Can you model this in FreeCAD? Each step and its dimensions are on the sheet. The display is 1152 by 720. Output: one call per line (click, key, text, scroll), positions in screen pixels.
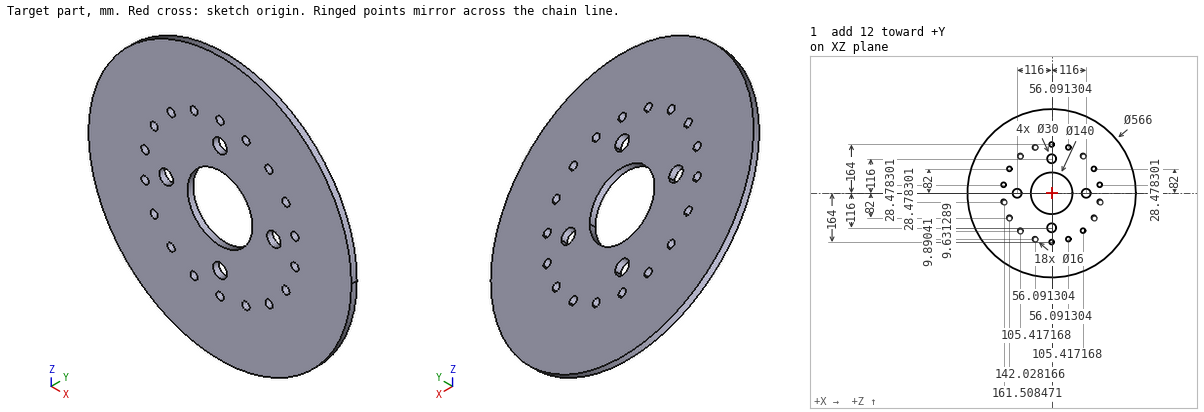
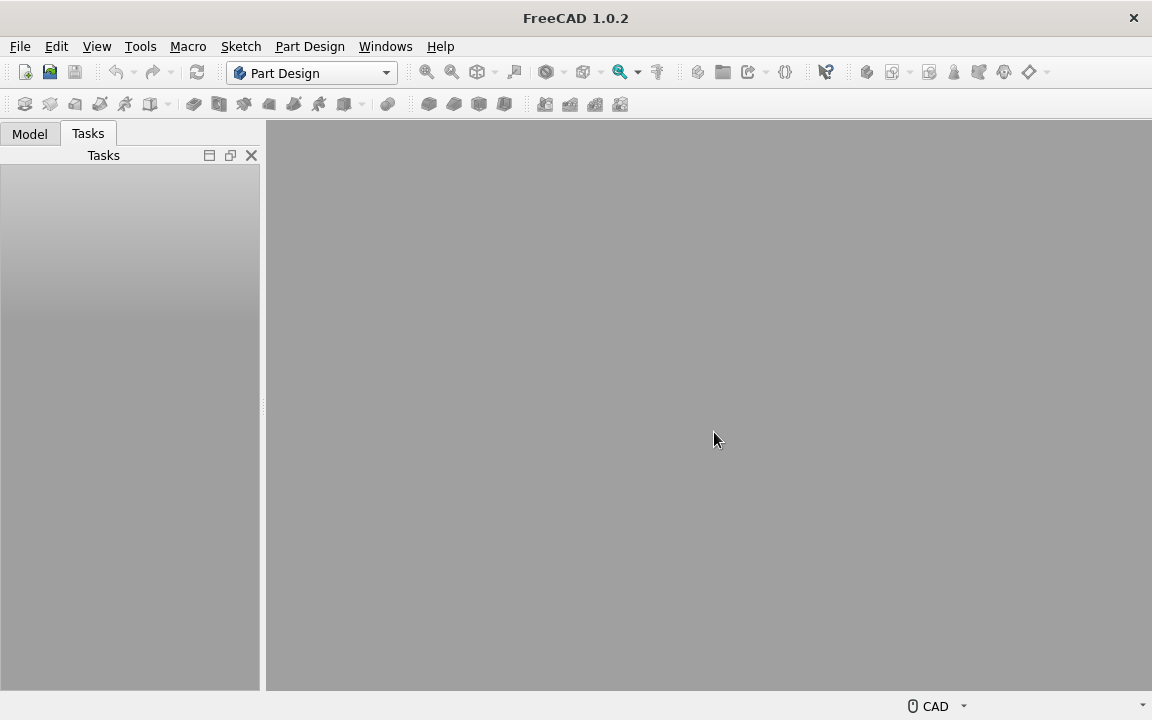
click(25, 72)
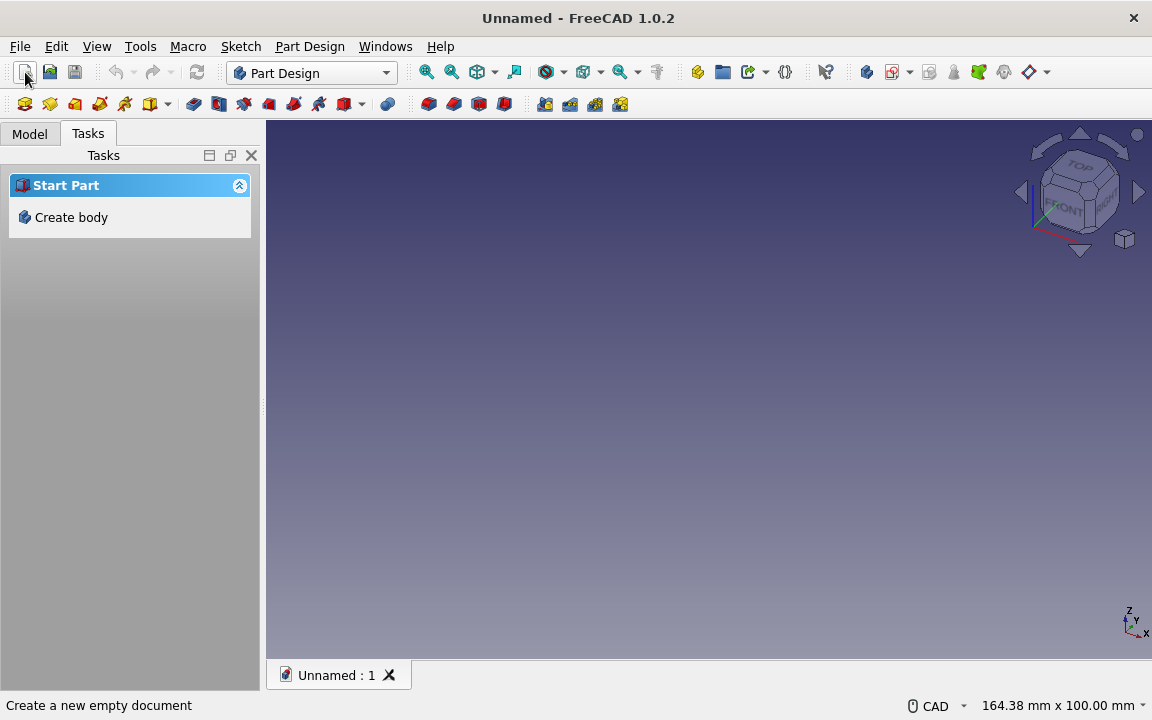
click(892, 72)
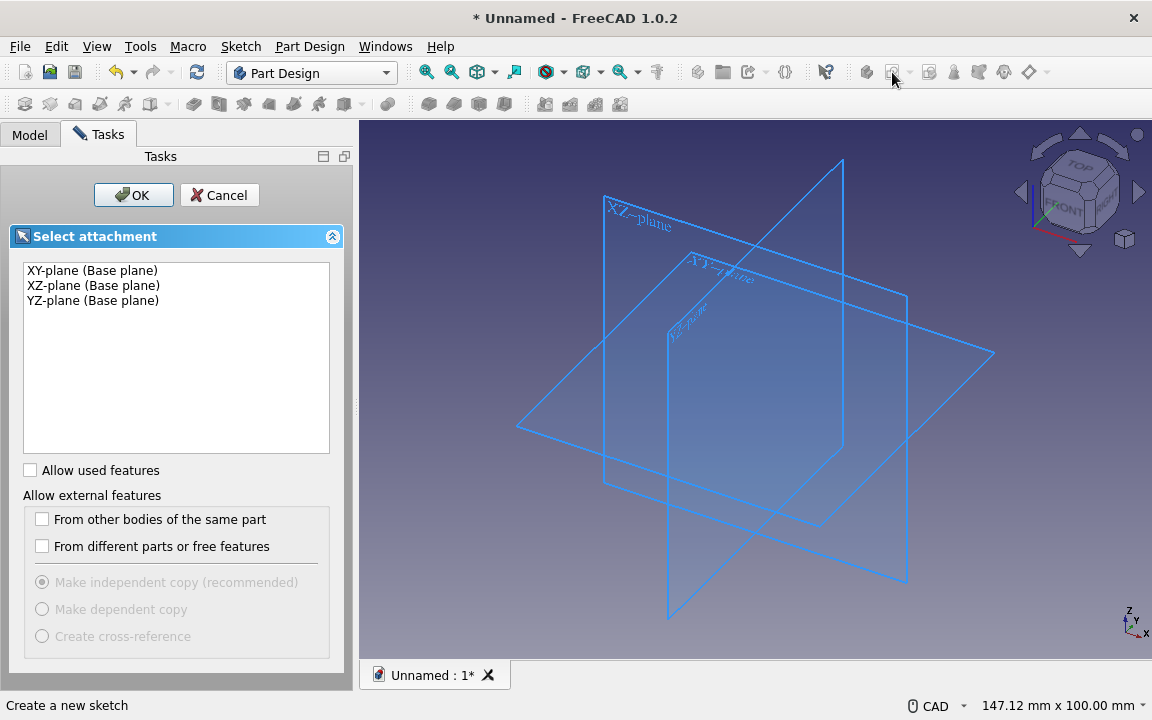
click(84, 286)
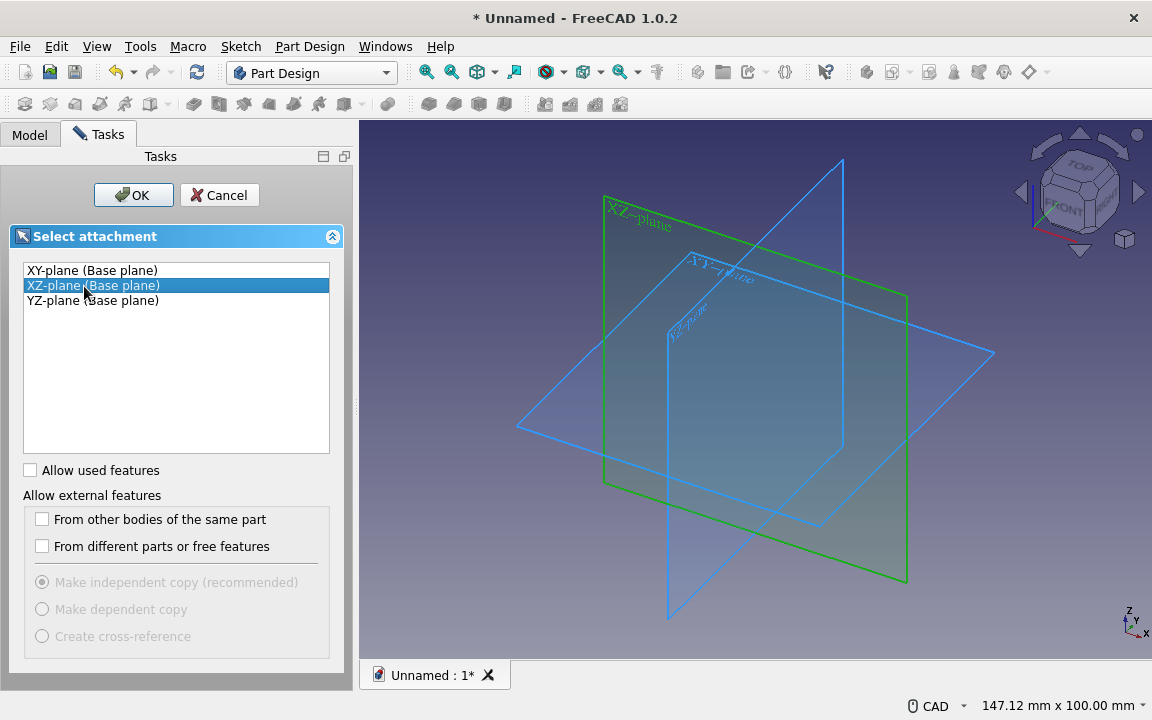
click(134, 195)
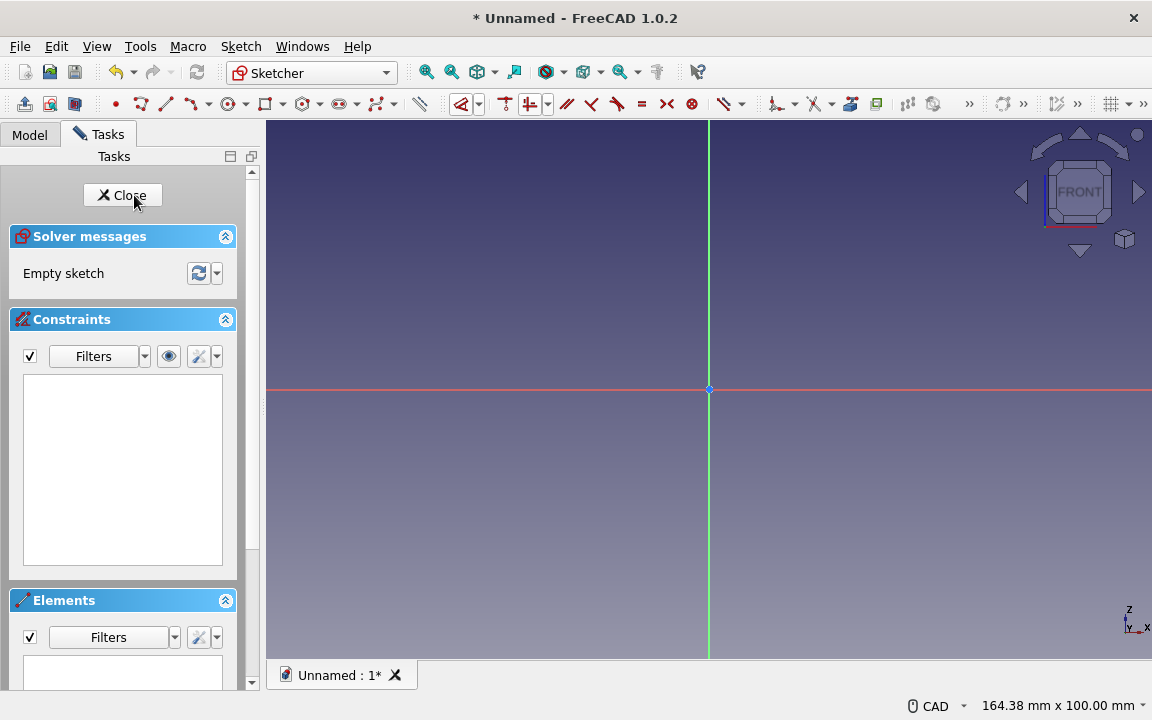
scroll(632, 390, down, 11)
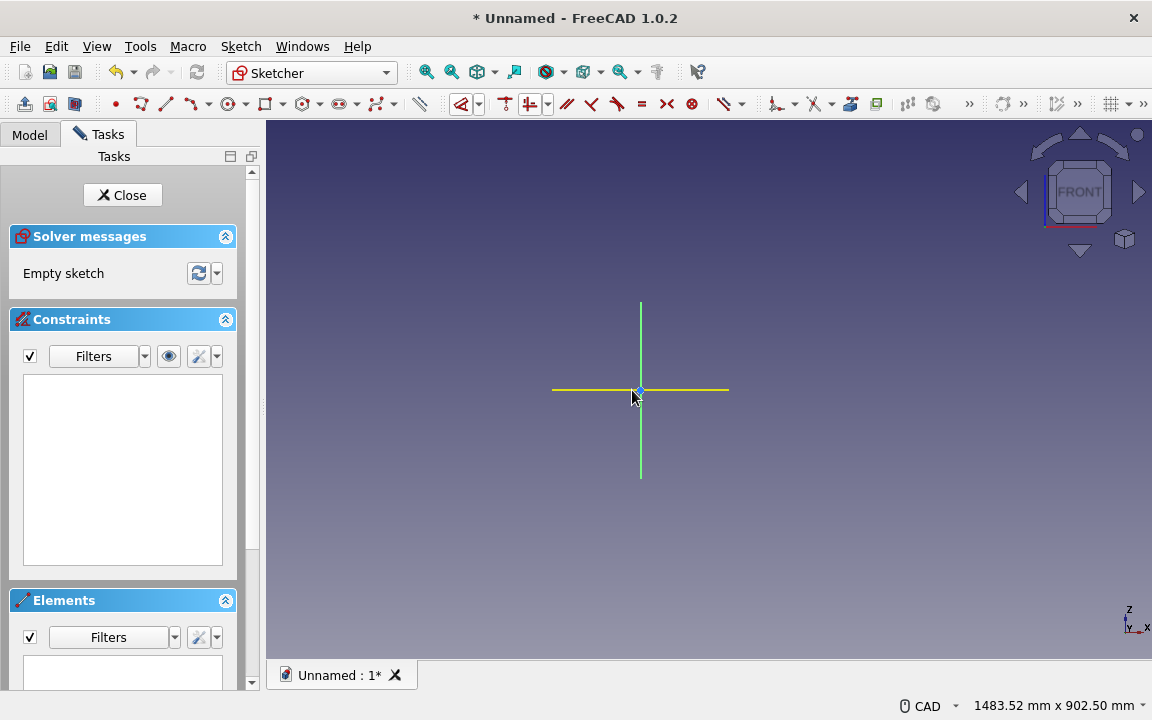
key(g)
key(c)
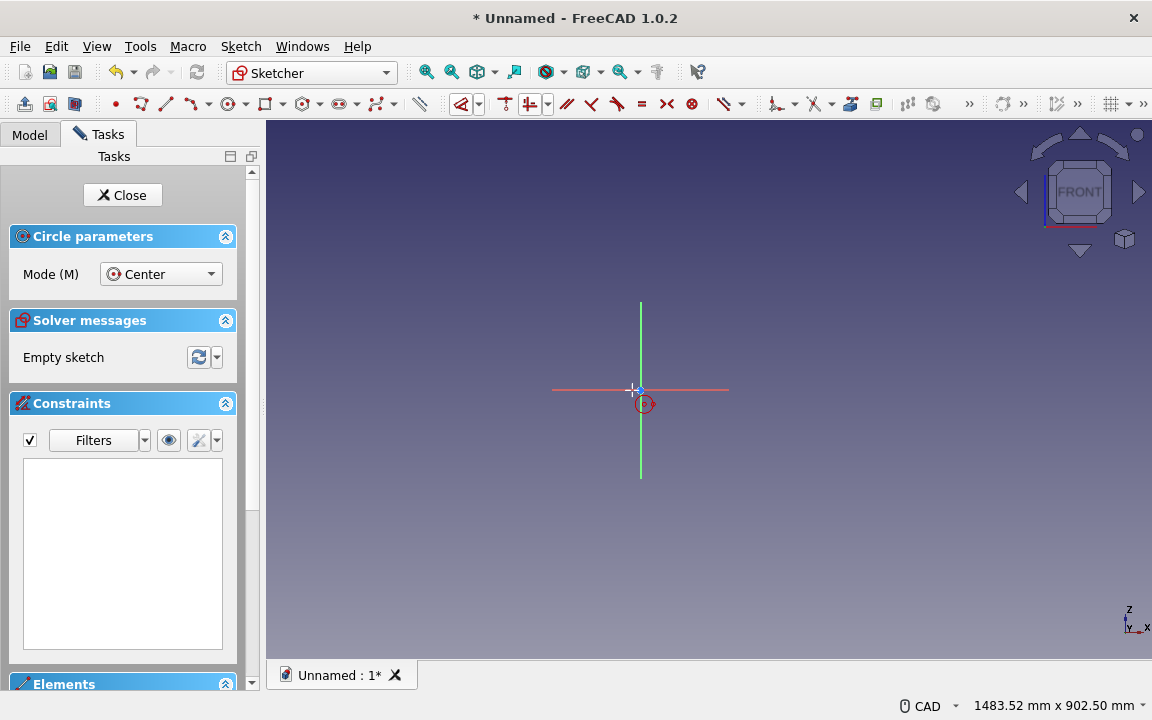
click(641, 390)
move(760, 271)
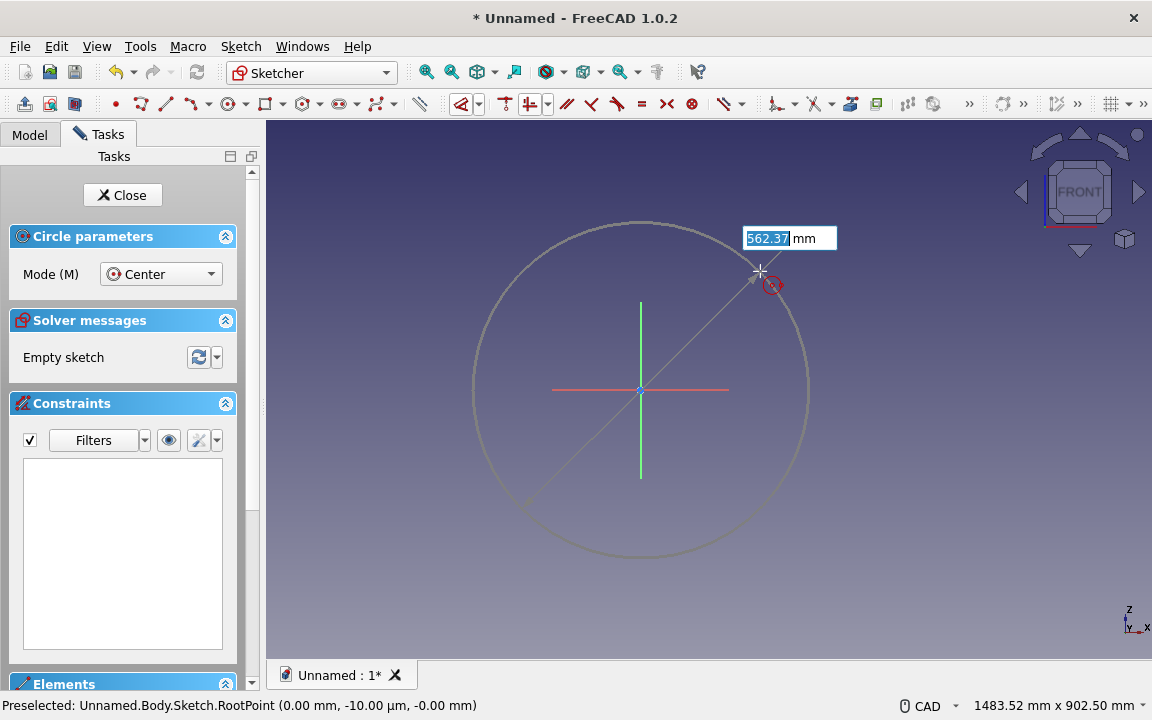
text(566)
key(Return)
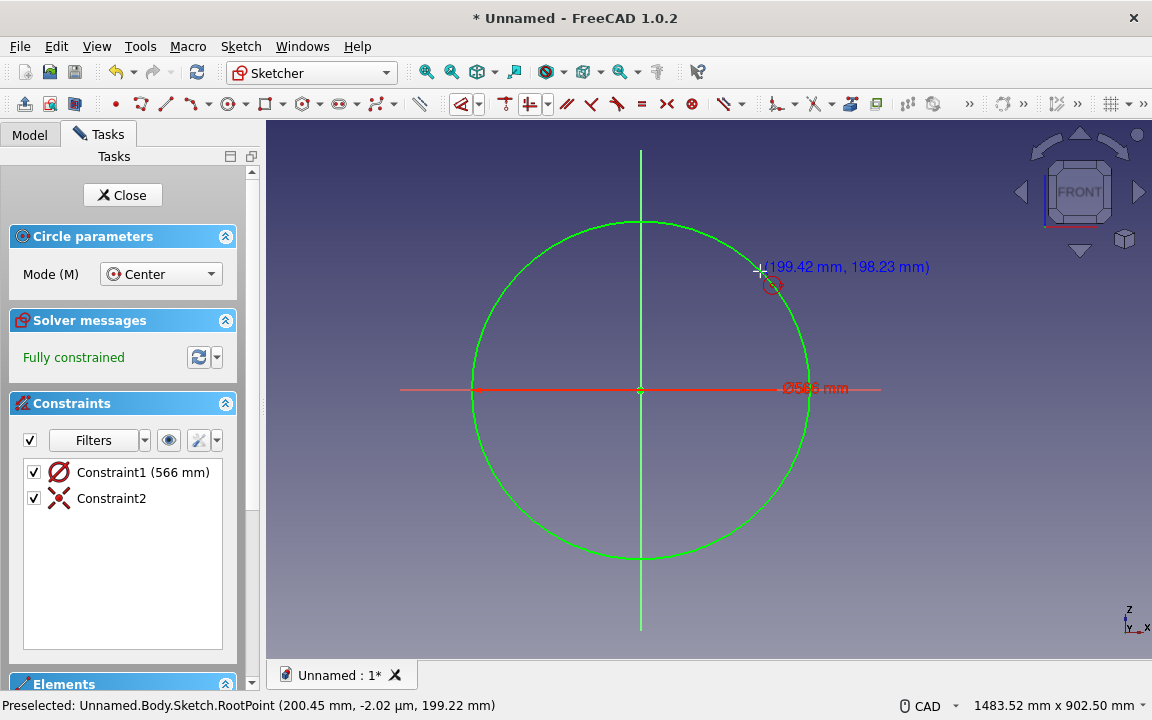
scroll(578, 465, up, 8)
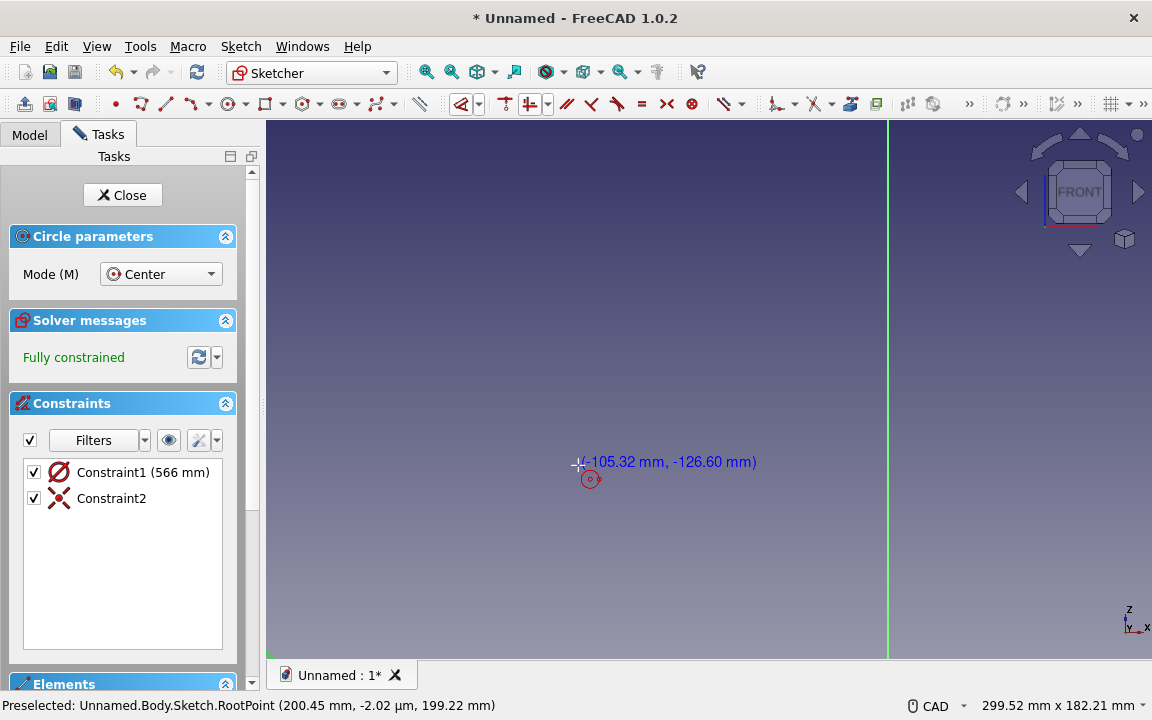
scroll(578, 465, down, 8)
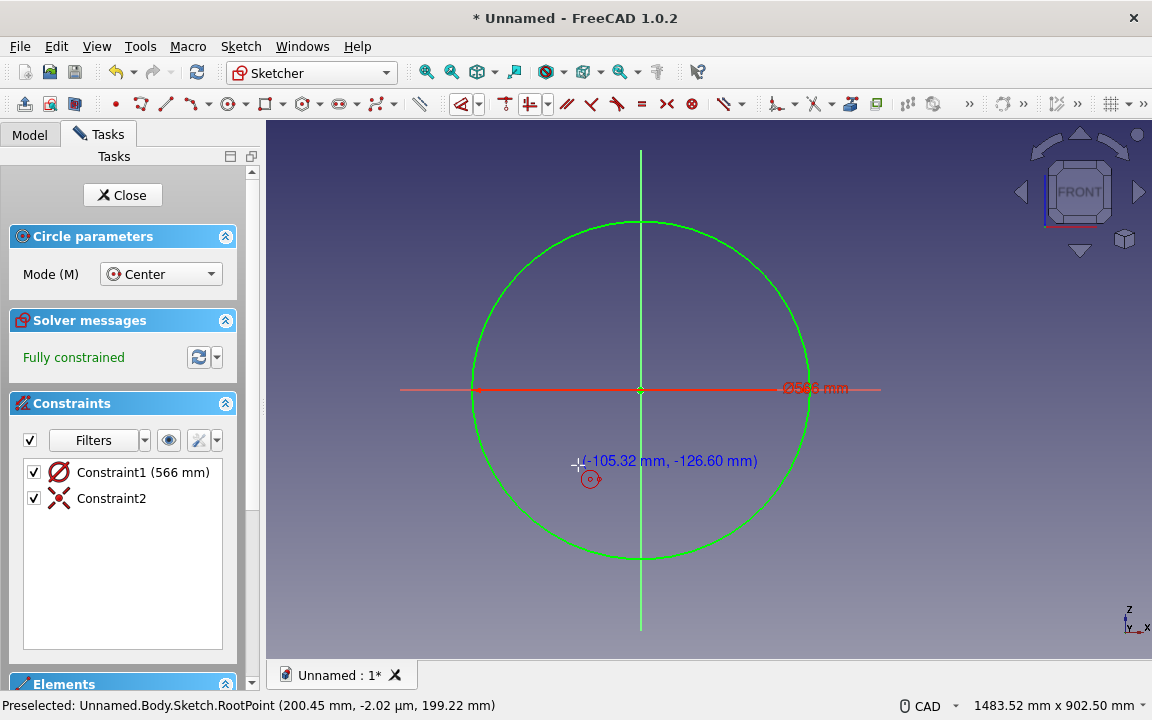
click(578, 465)
move(581, 462)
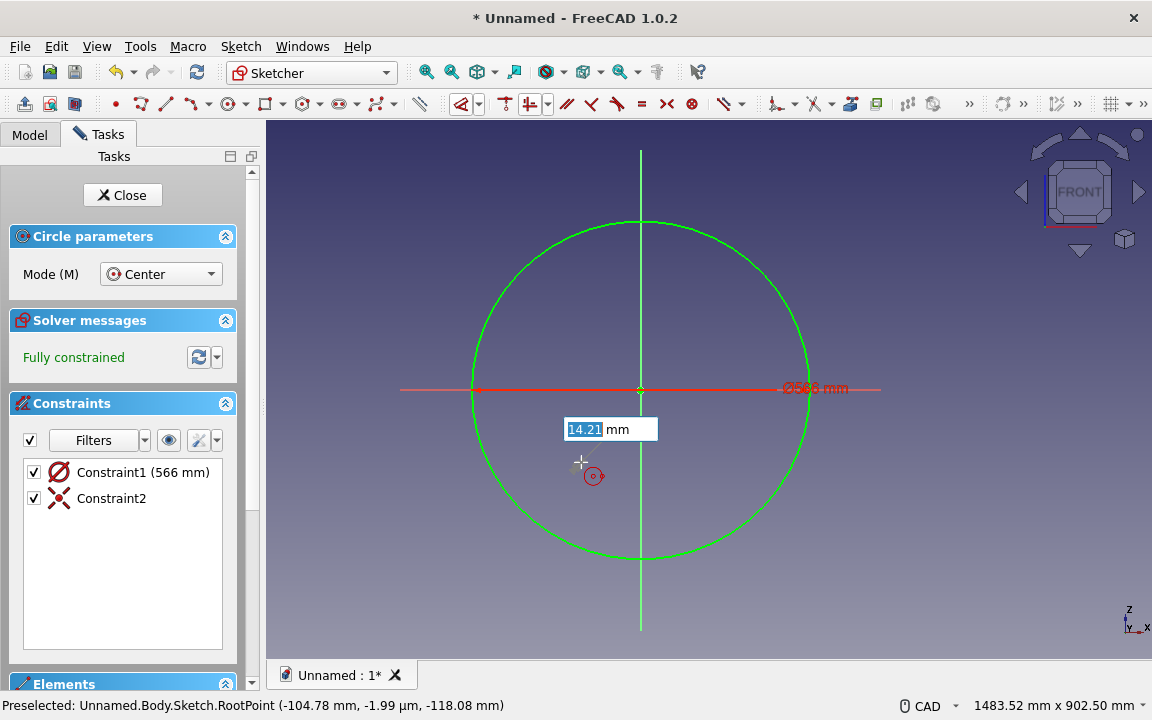
text(16)
key(Return)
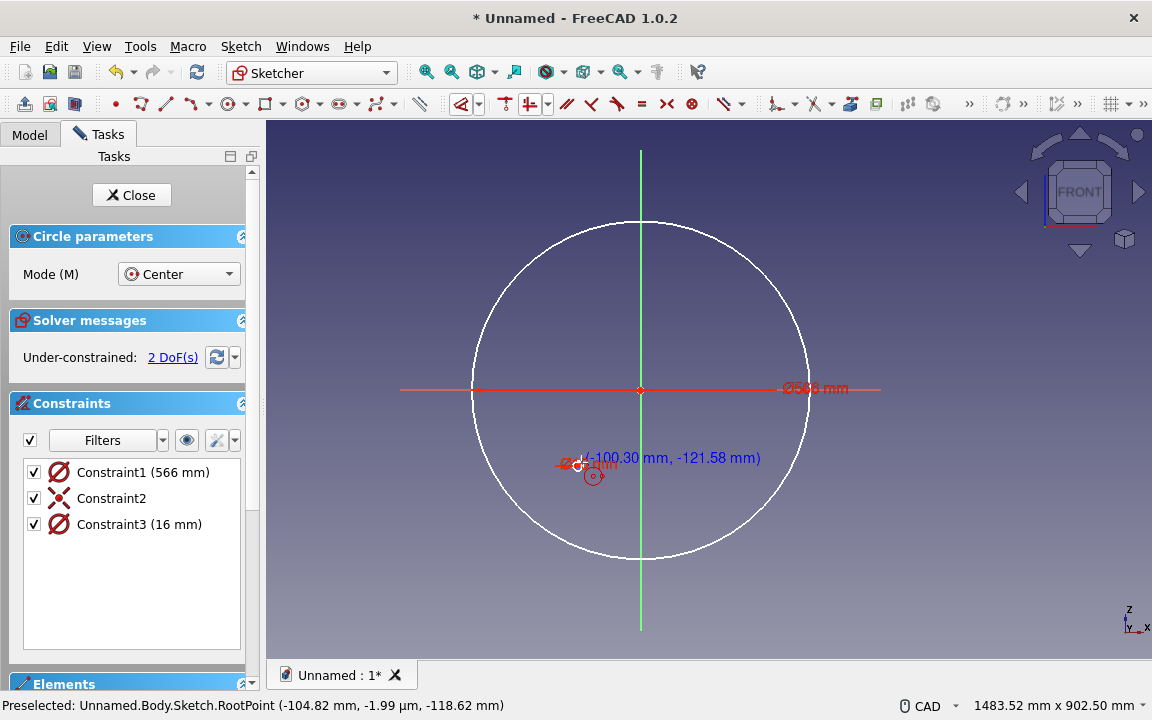
scroll(556, 439, up, 8)